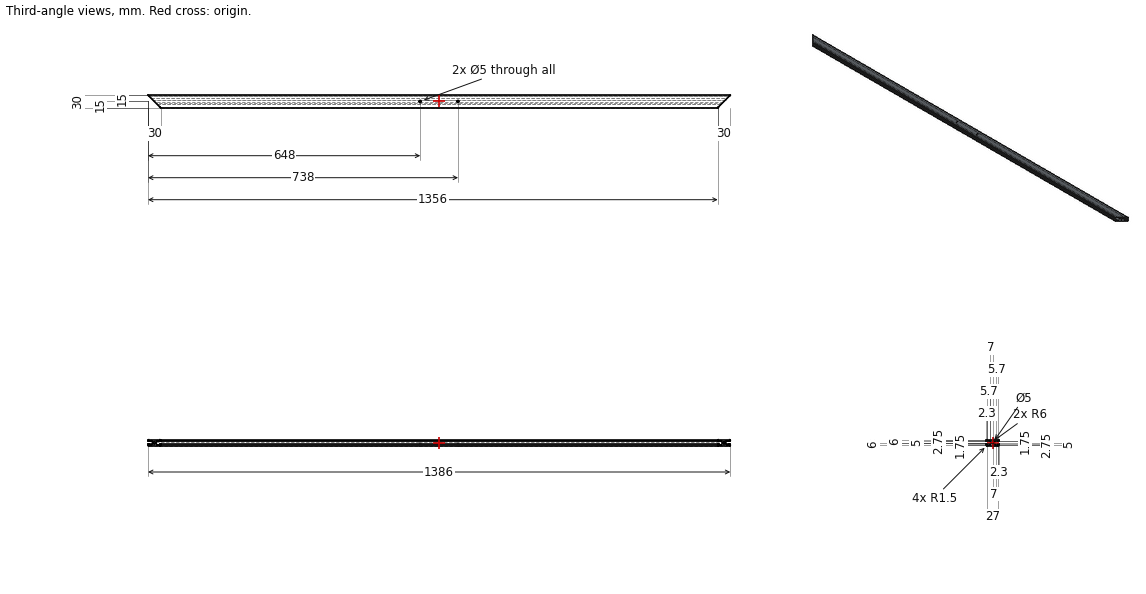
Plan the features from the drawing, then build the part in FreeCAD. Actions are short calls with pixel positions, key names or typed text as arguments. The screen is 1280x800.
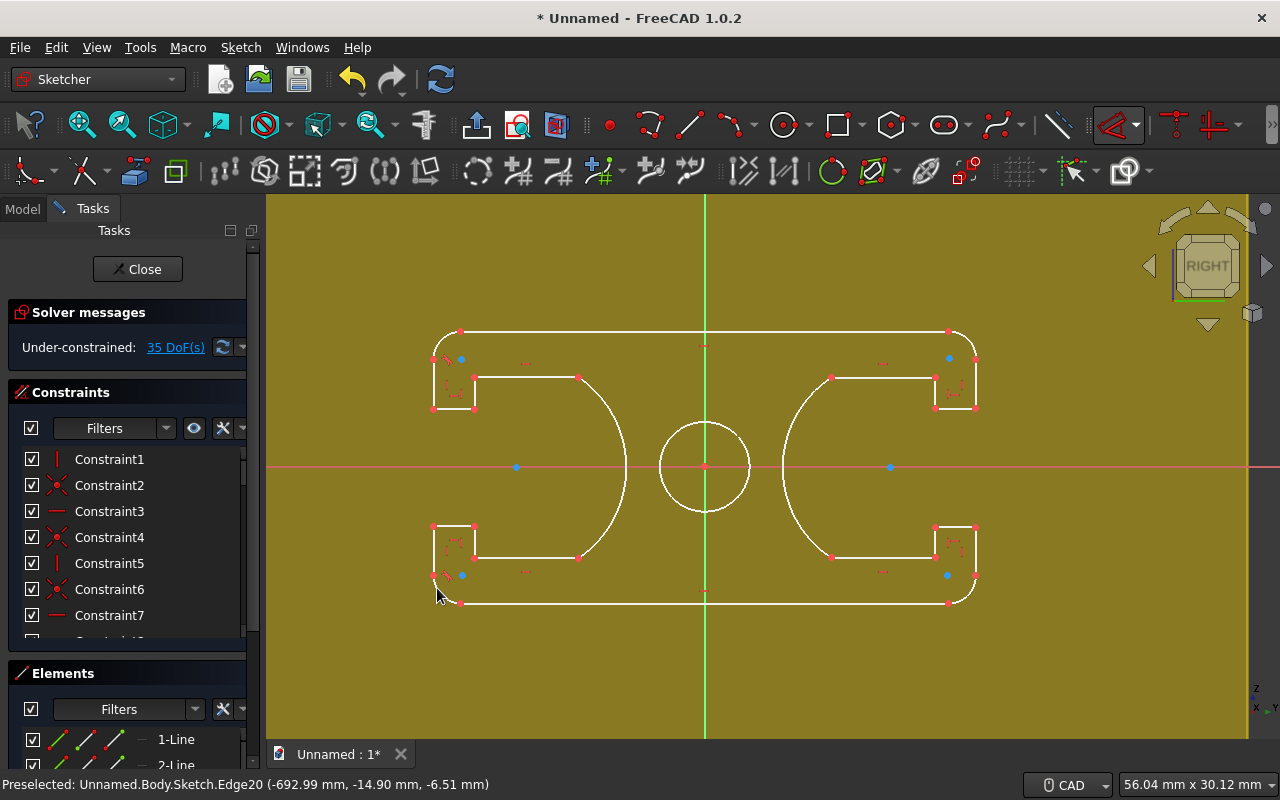
click(607, 604)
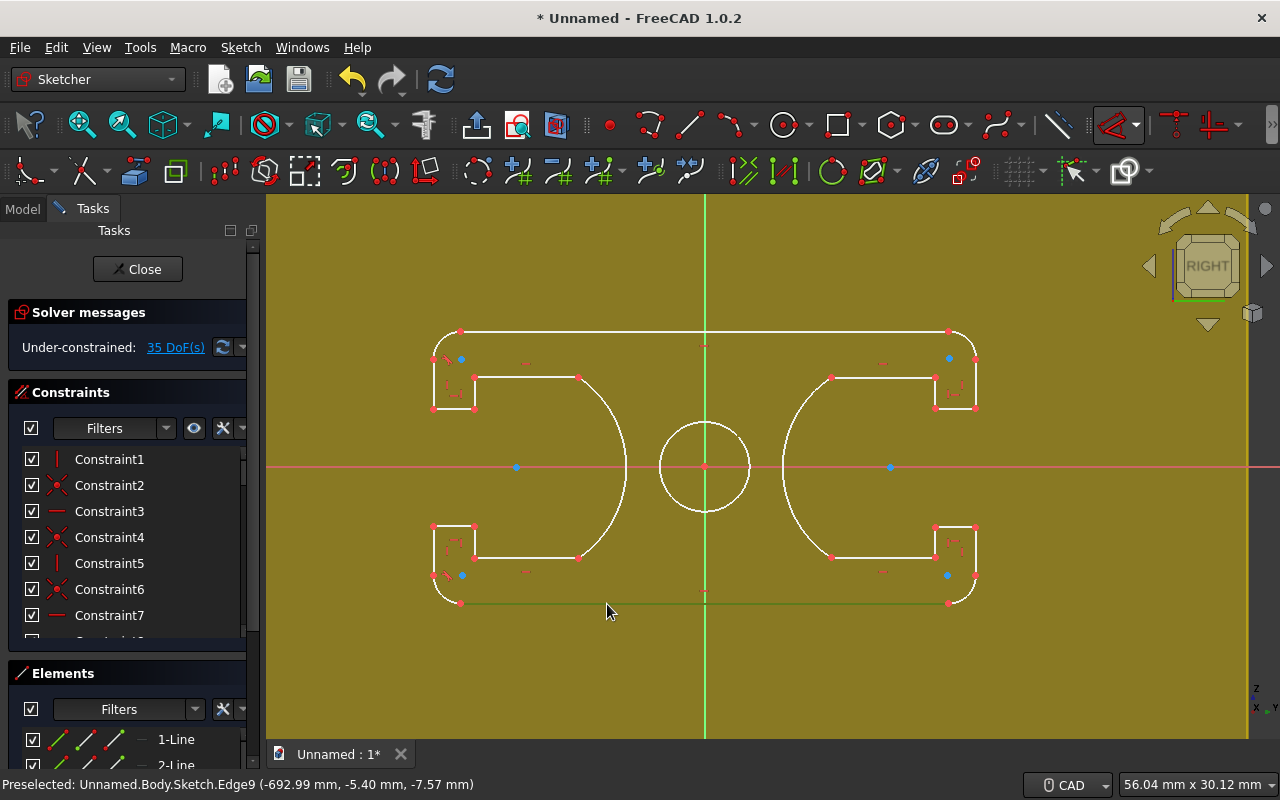
click(437, 588)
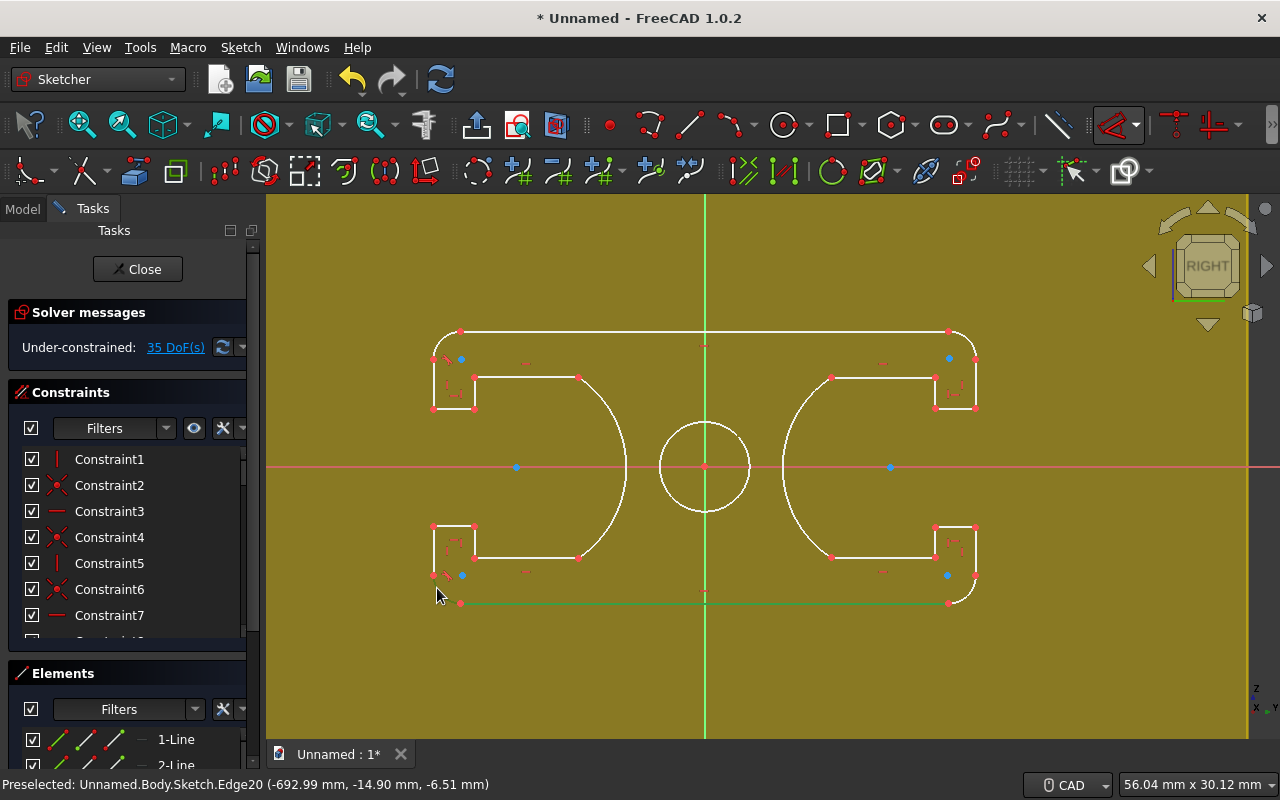
key(t)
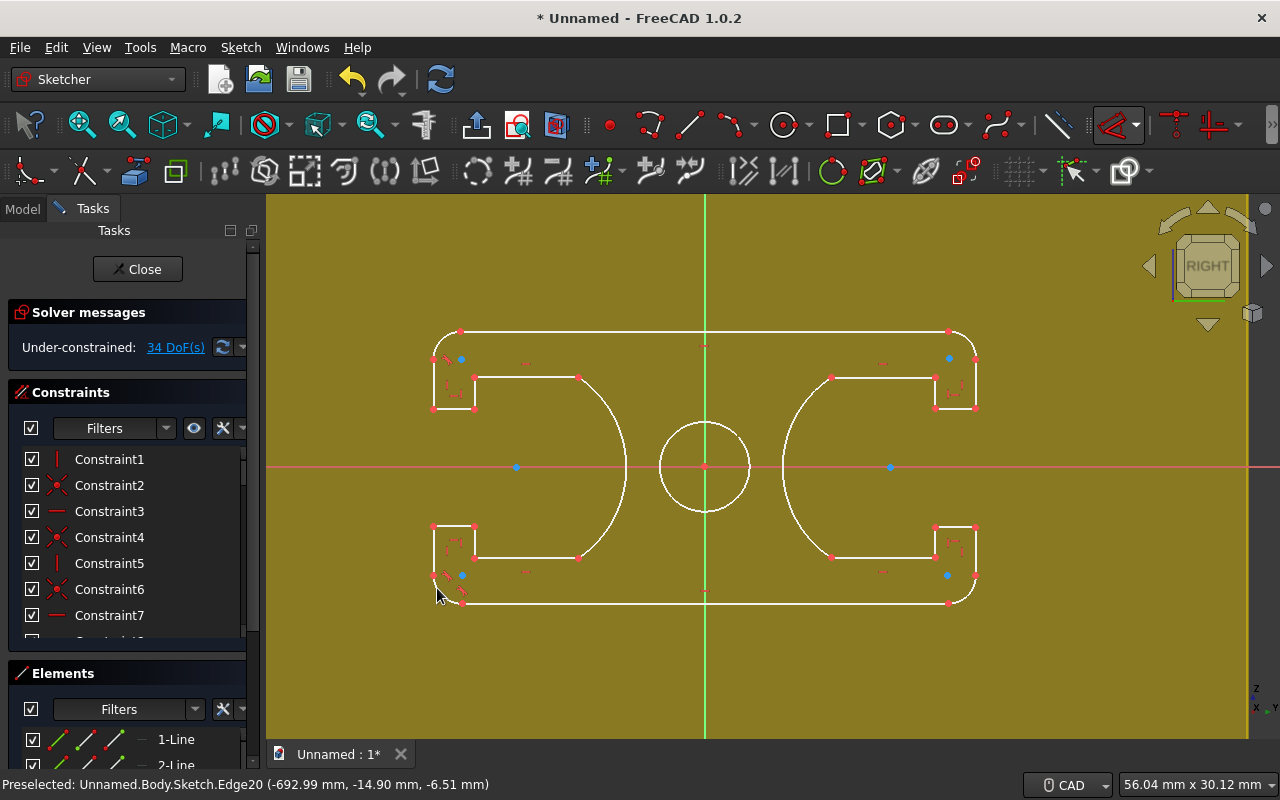
click(608, 604)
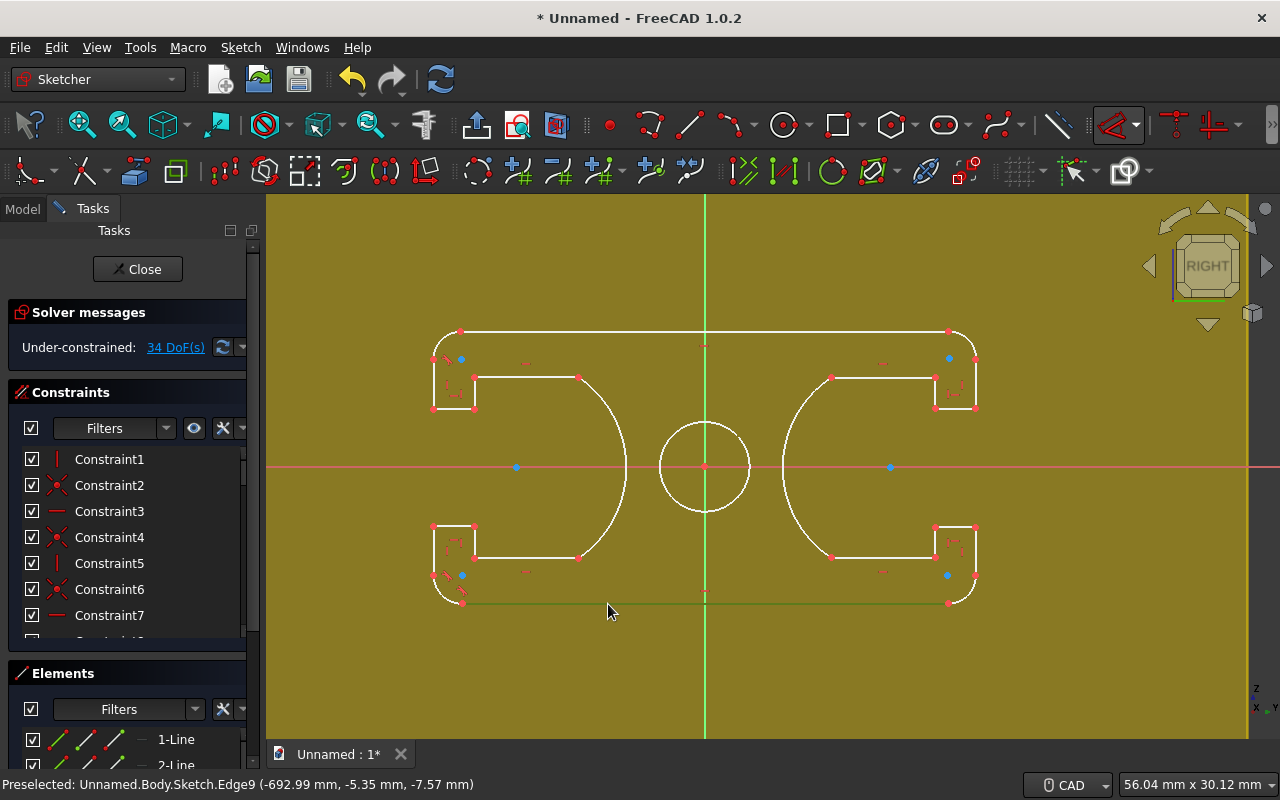
click(961, 600)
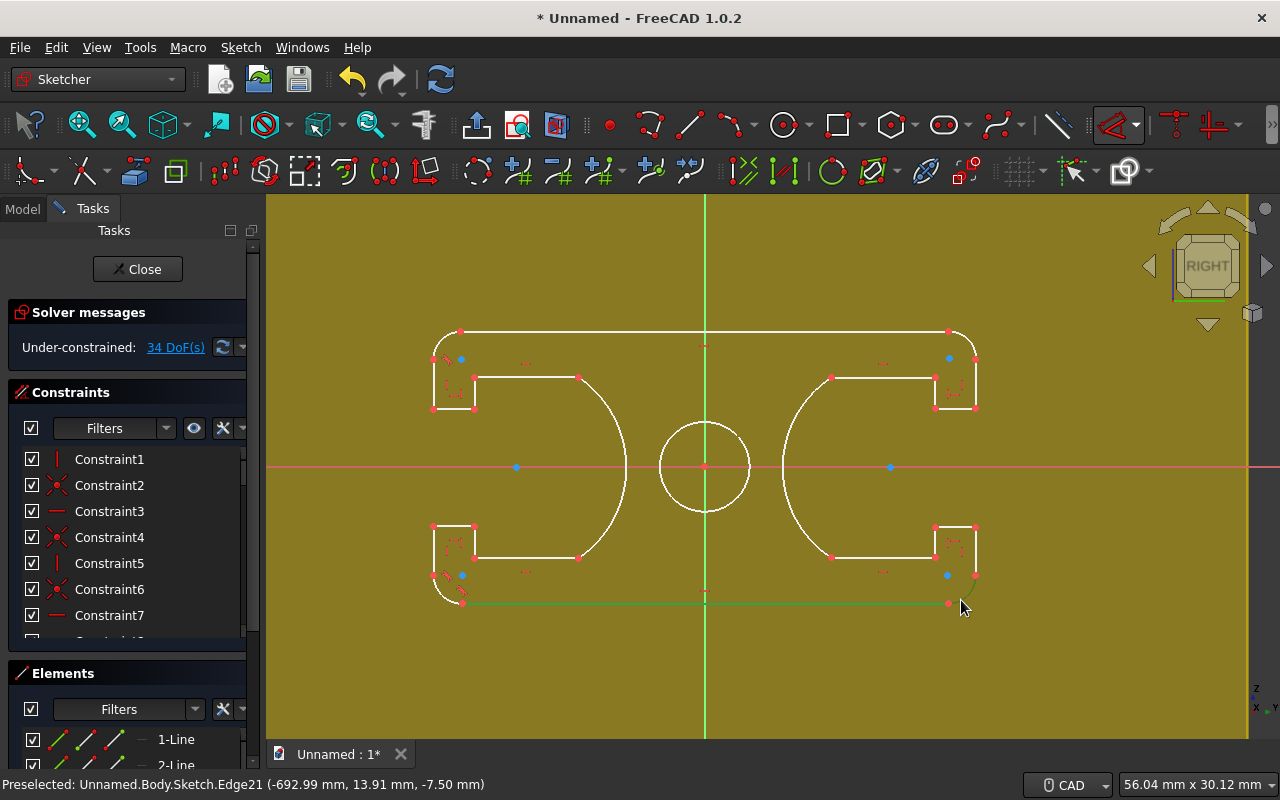
key(t)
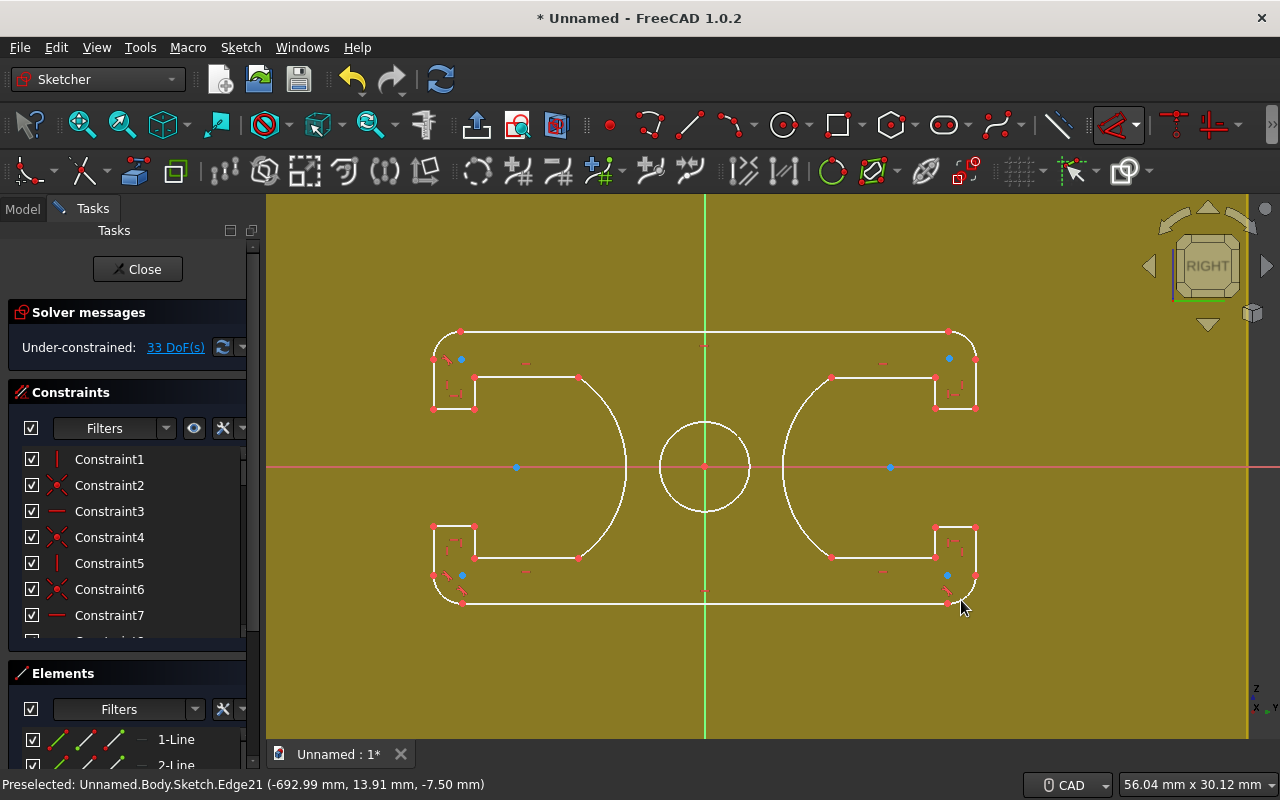
click(976, 561)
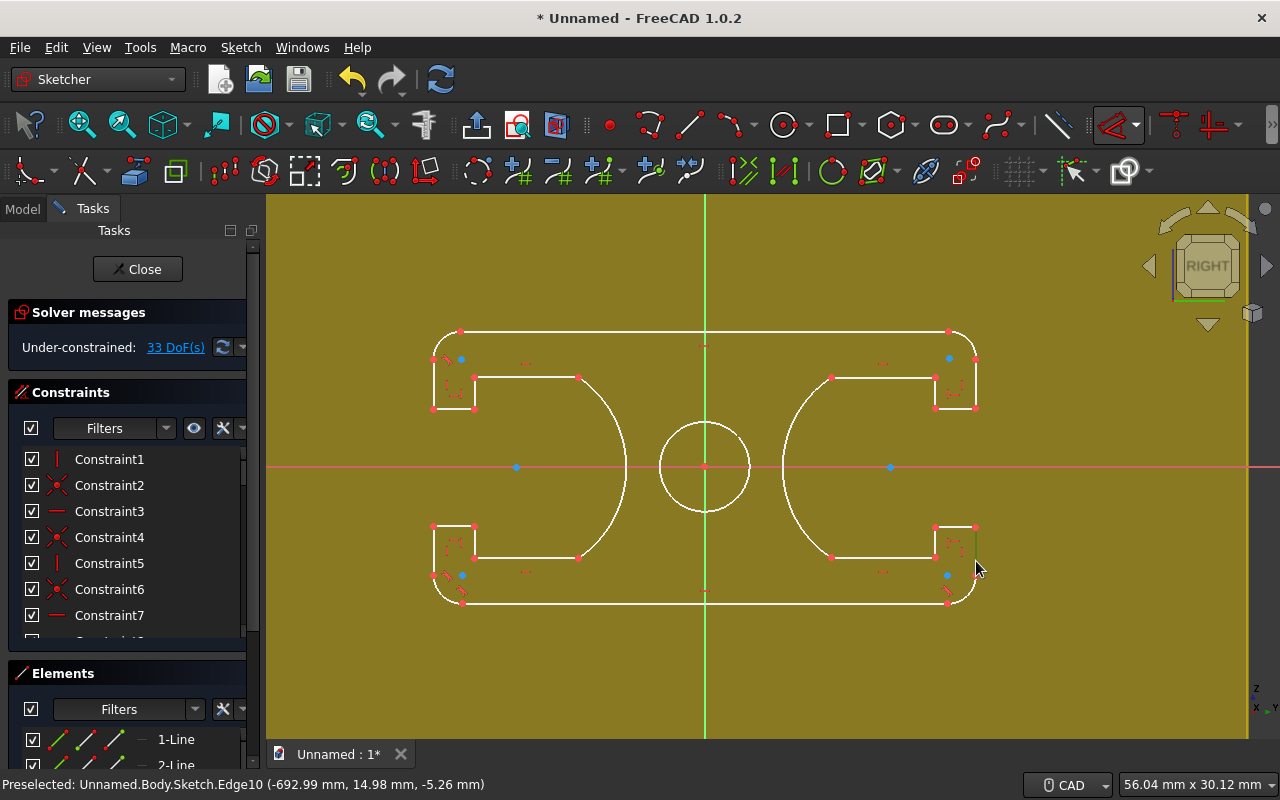
click(960, 601)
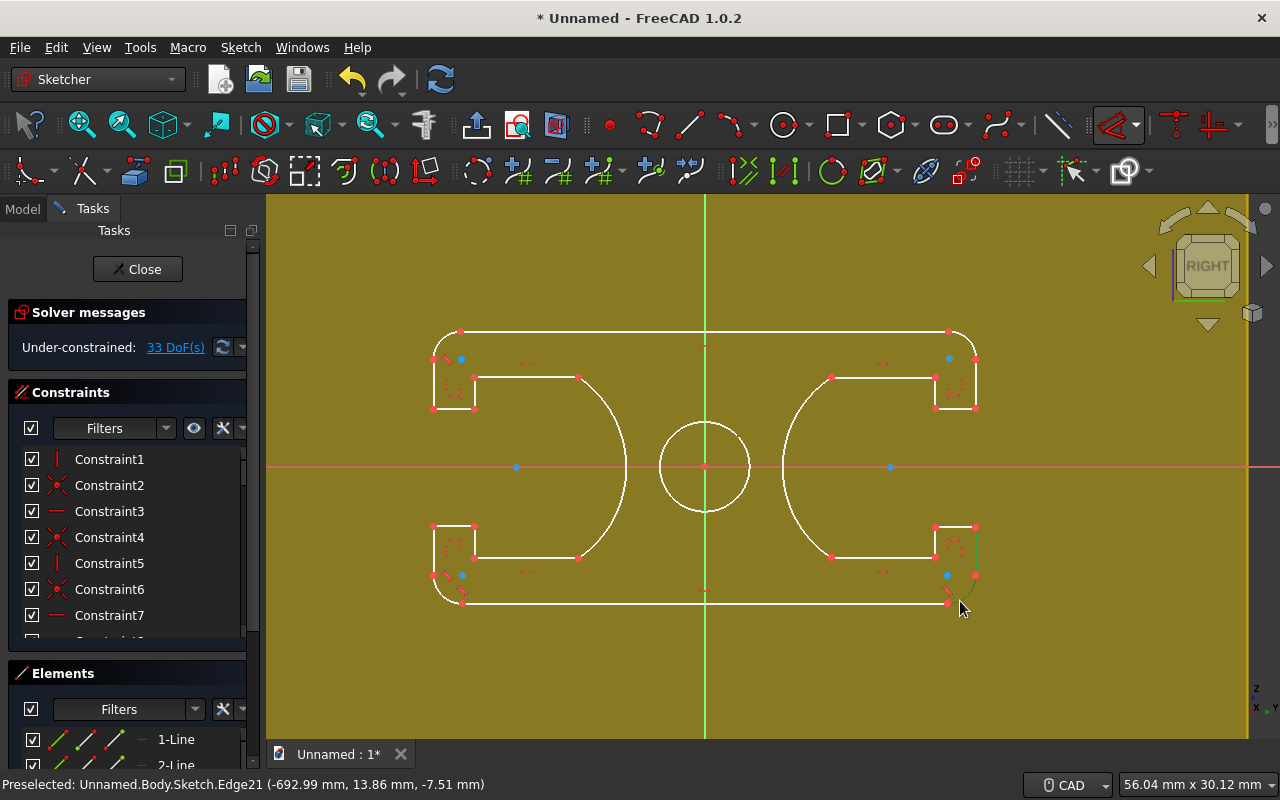
key(t)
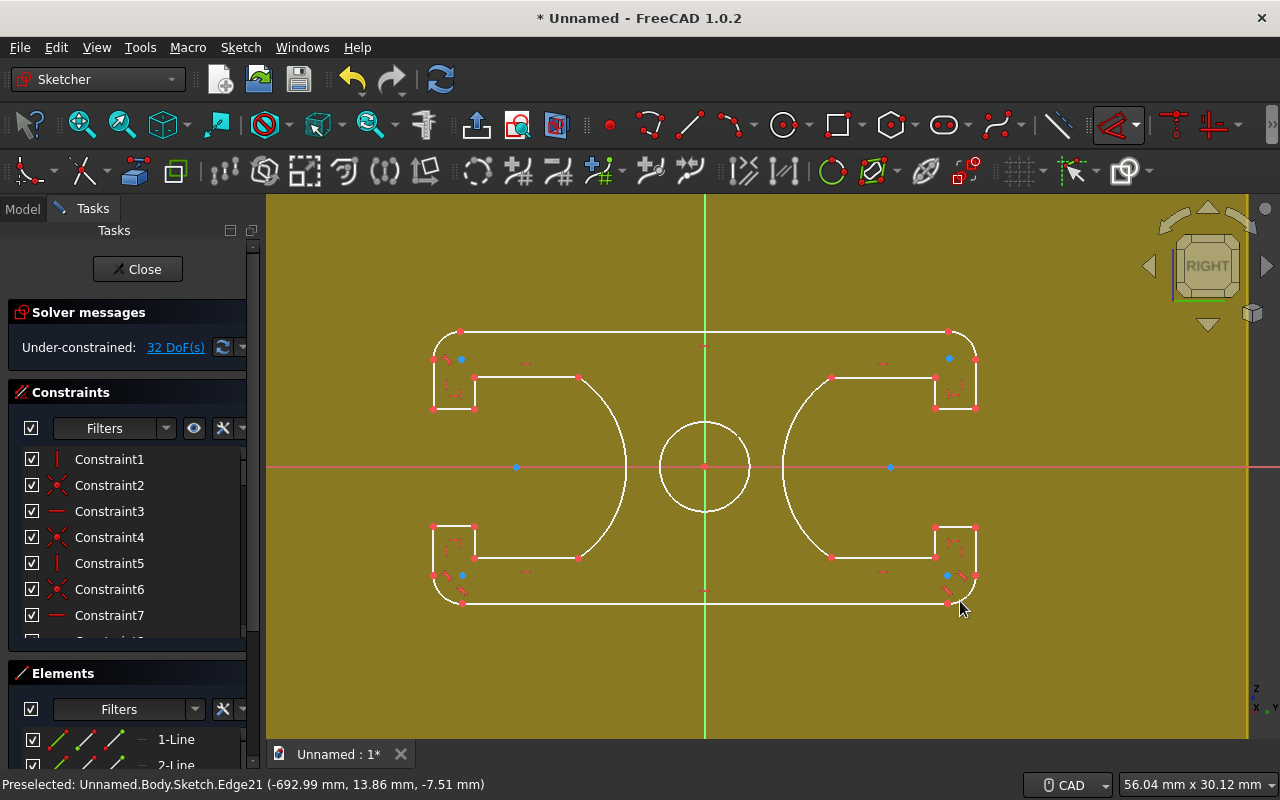
click(976, 394)